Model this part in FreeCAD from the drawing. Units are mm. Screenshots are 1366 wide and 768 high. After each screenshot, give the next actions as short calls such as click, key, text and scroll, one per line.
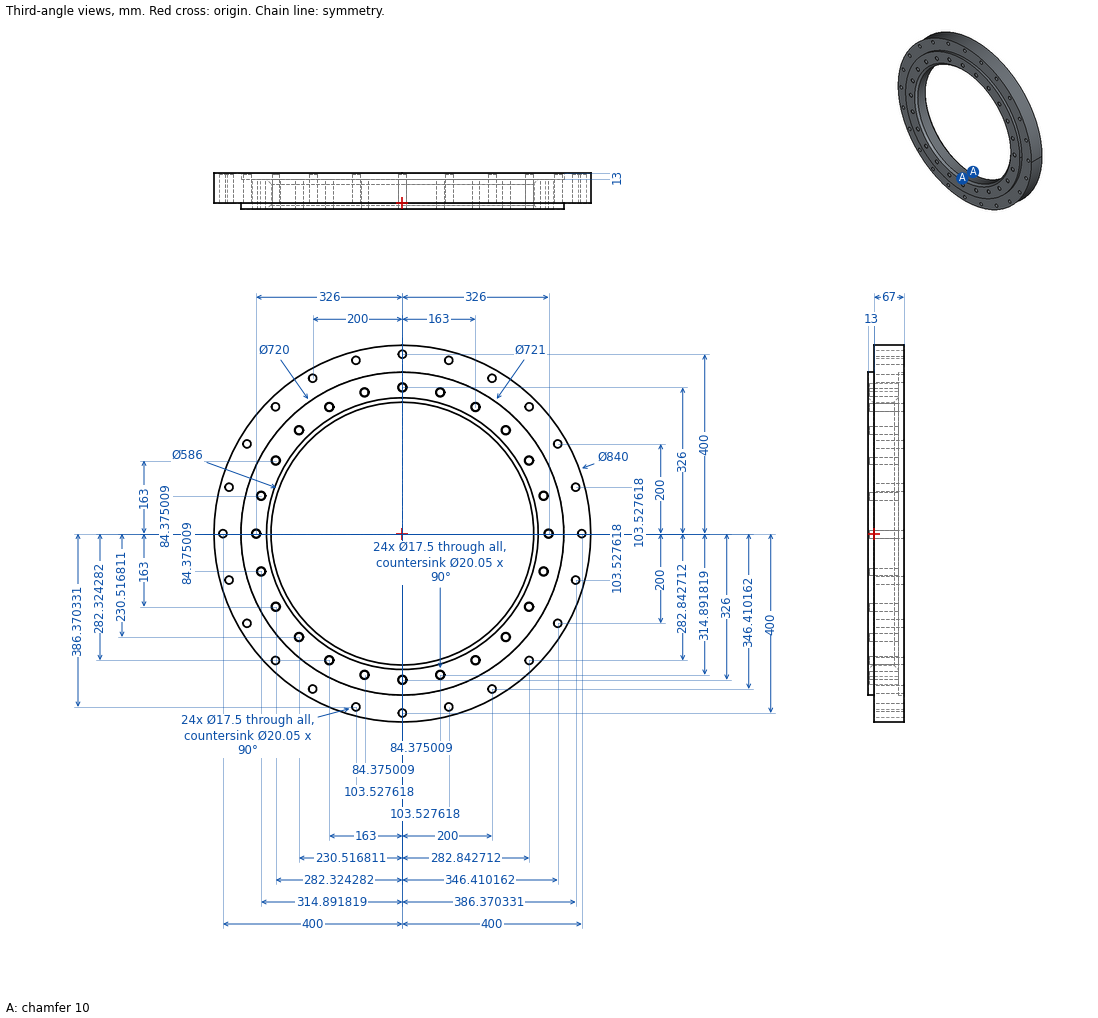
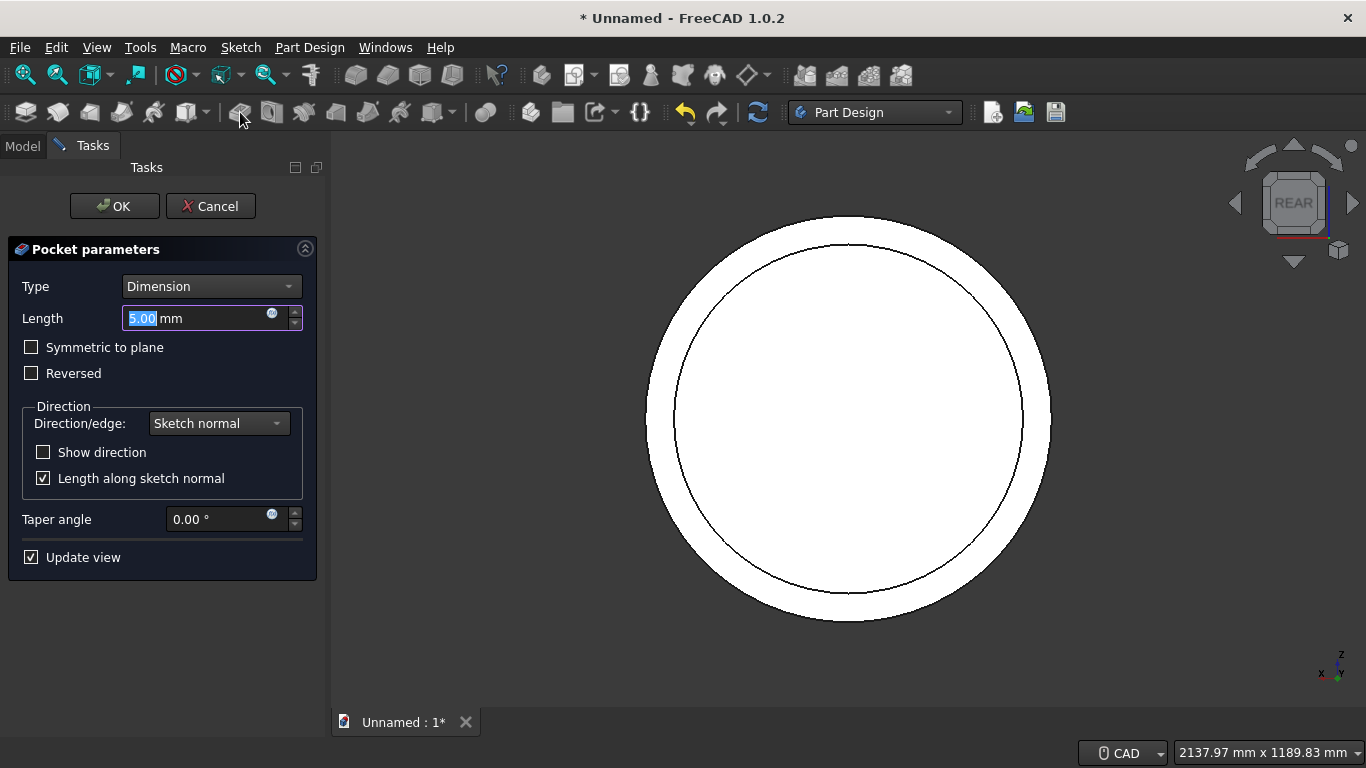
text(13)
key(Tab)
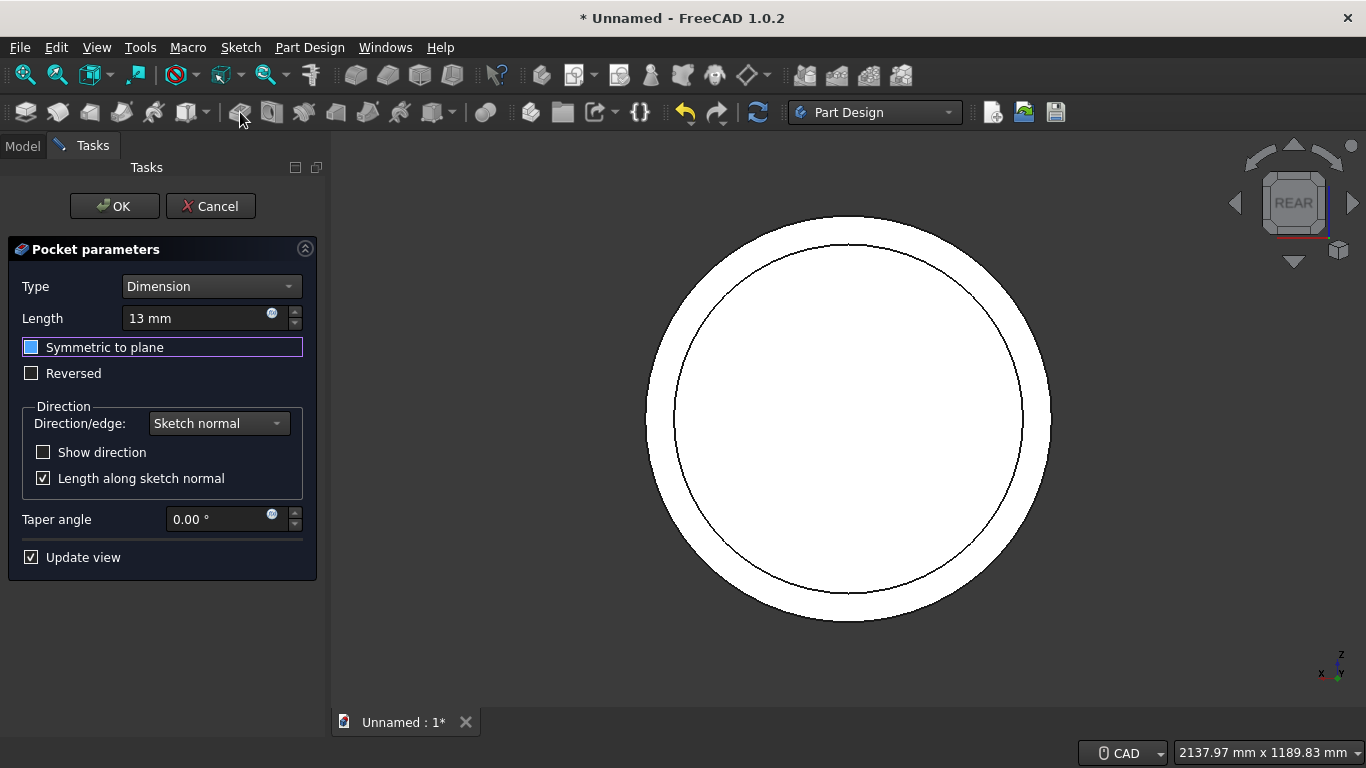
click(115, 206)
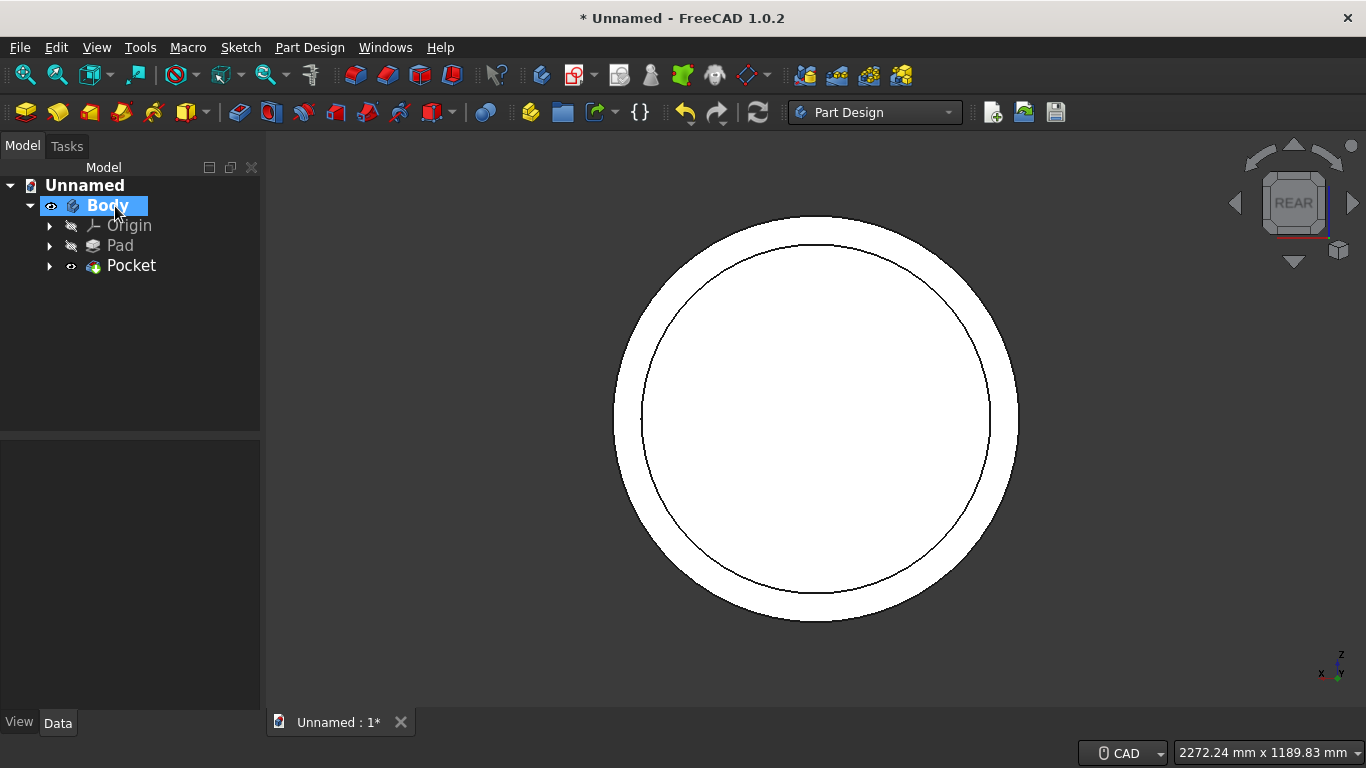
click(574, 76)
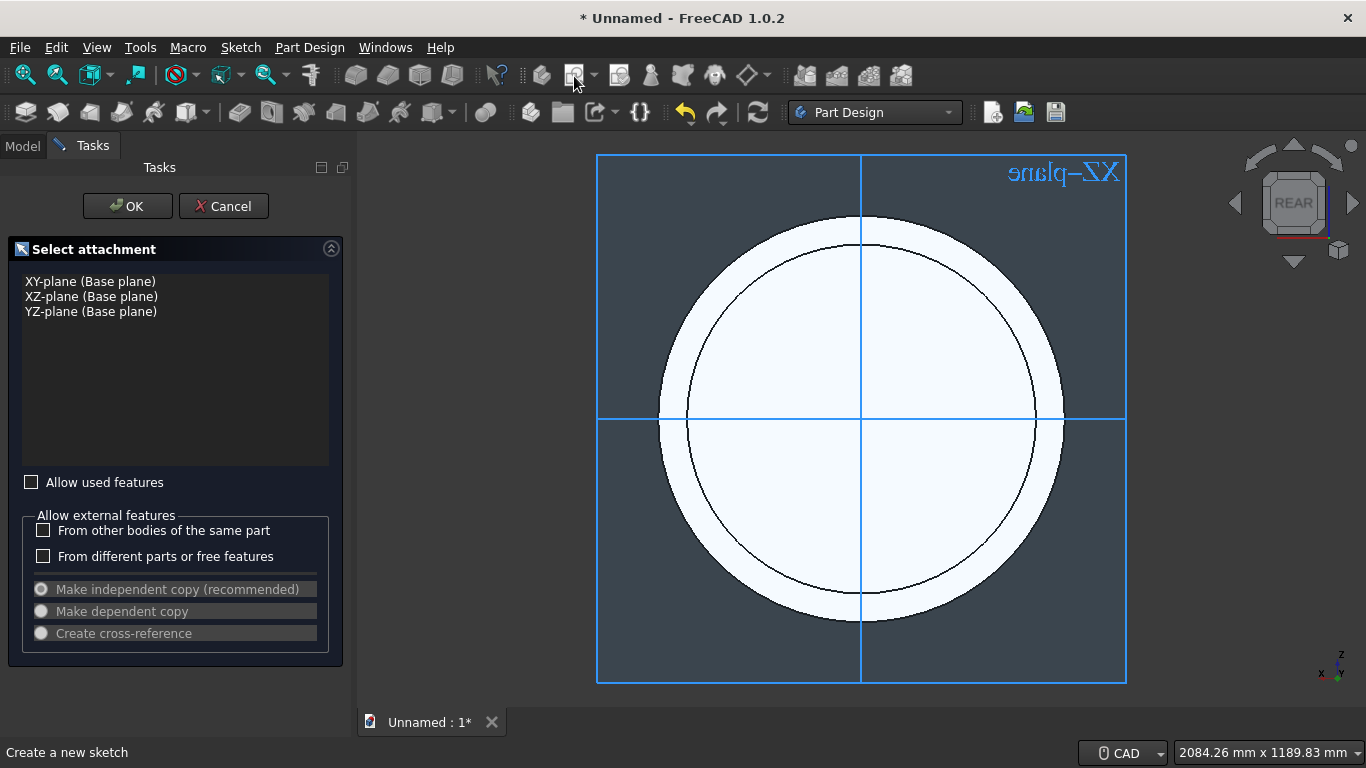
click(82, 296)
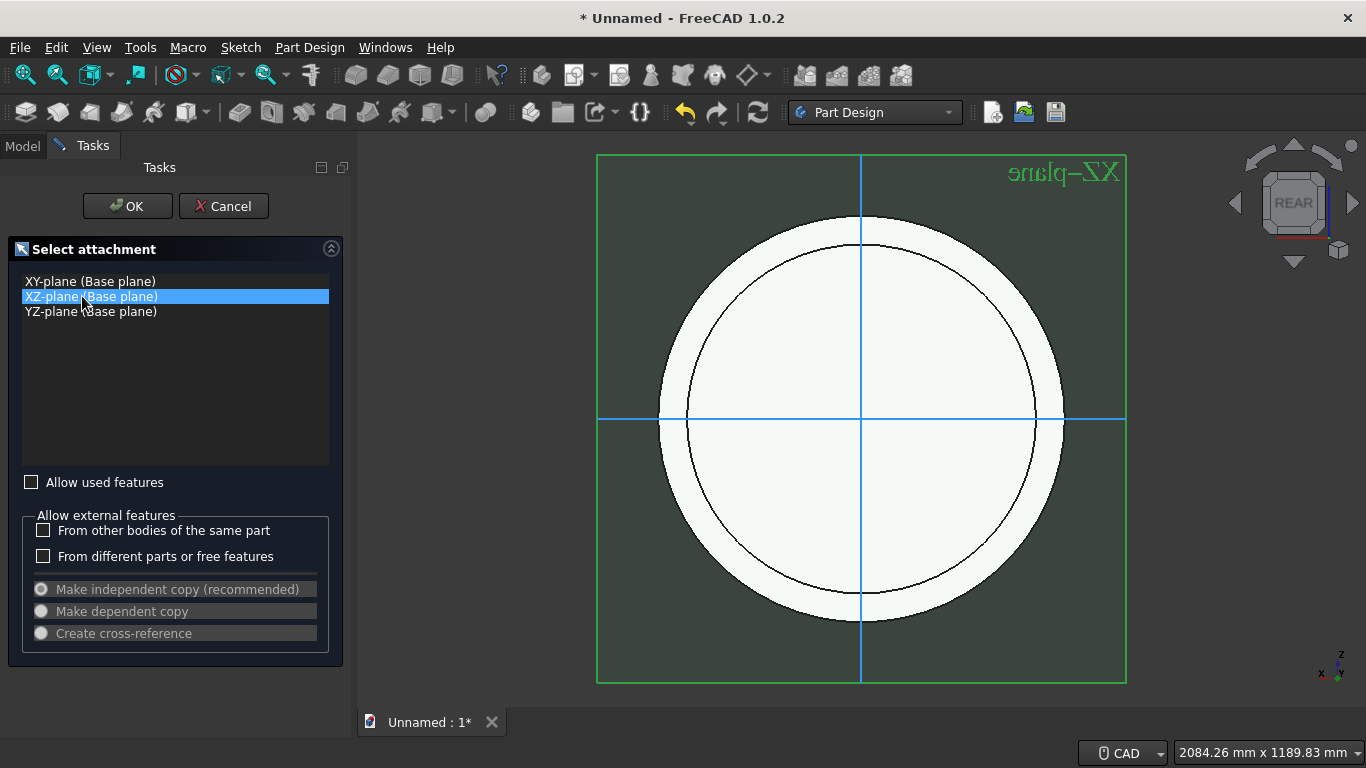
click(128, 206)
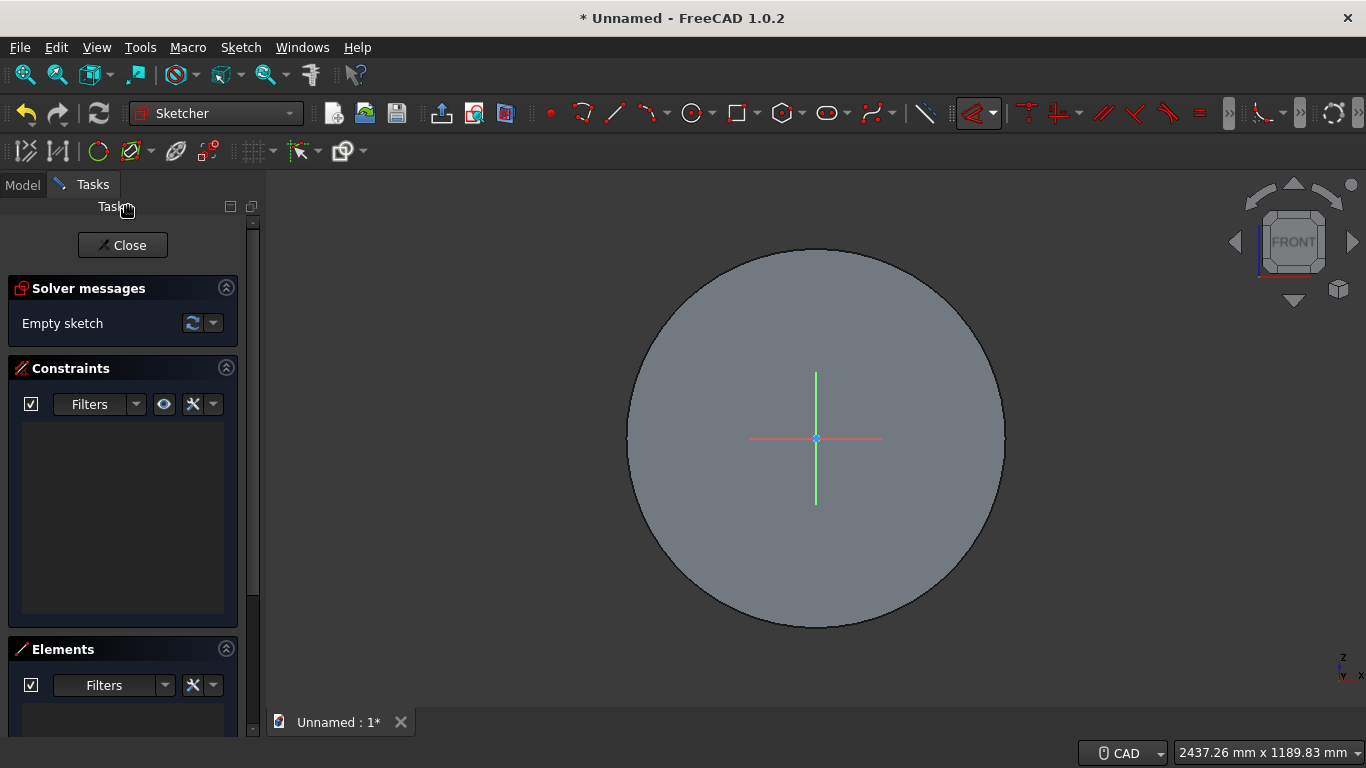
click(692, 114)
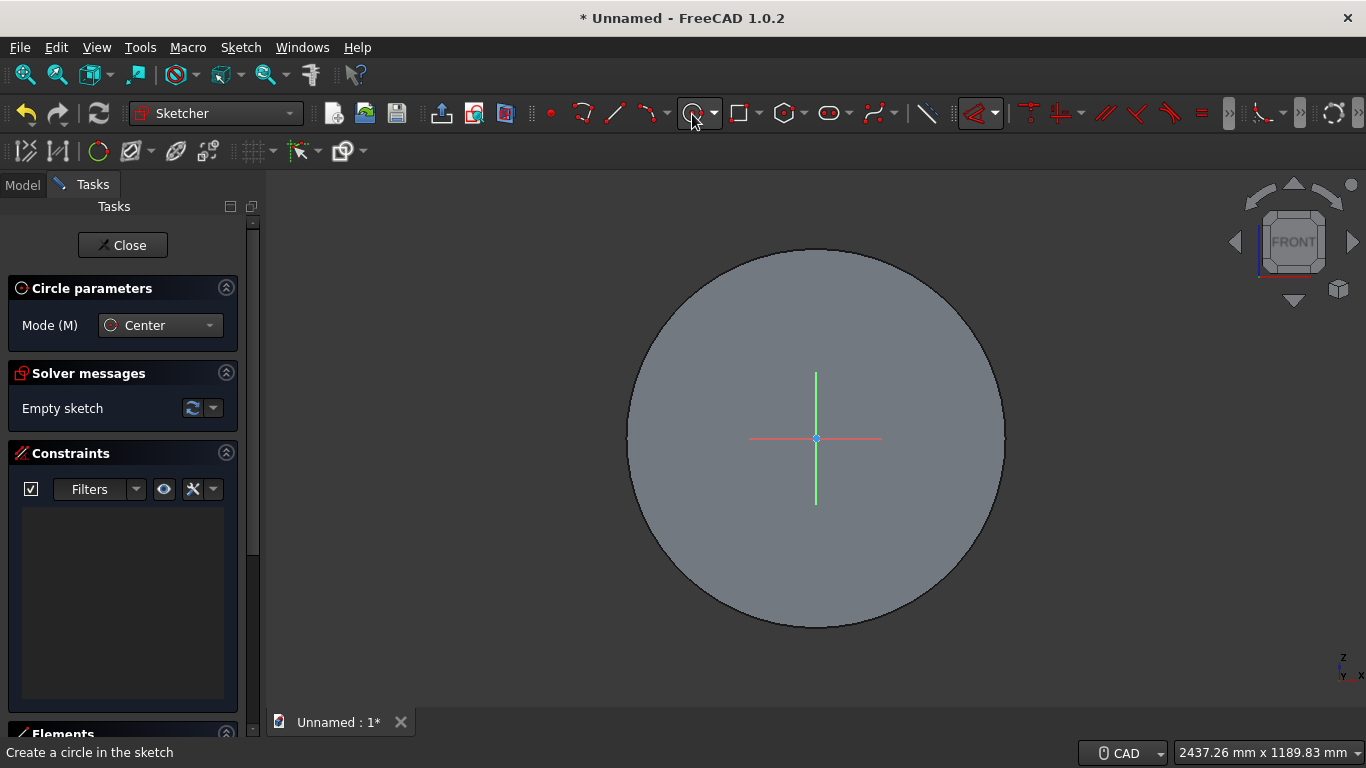
click(816, 439)
click(931, 324)
key(Escape)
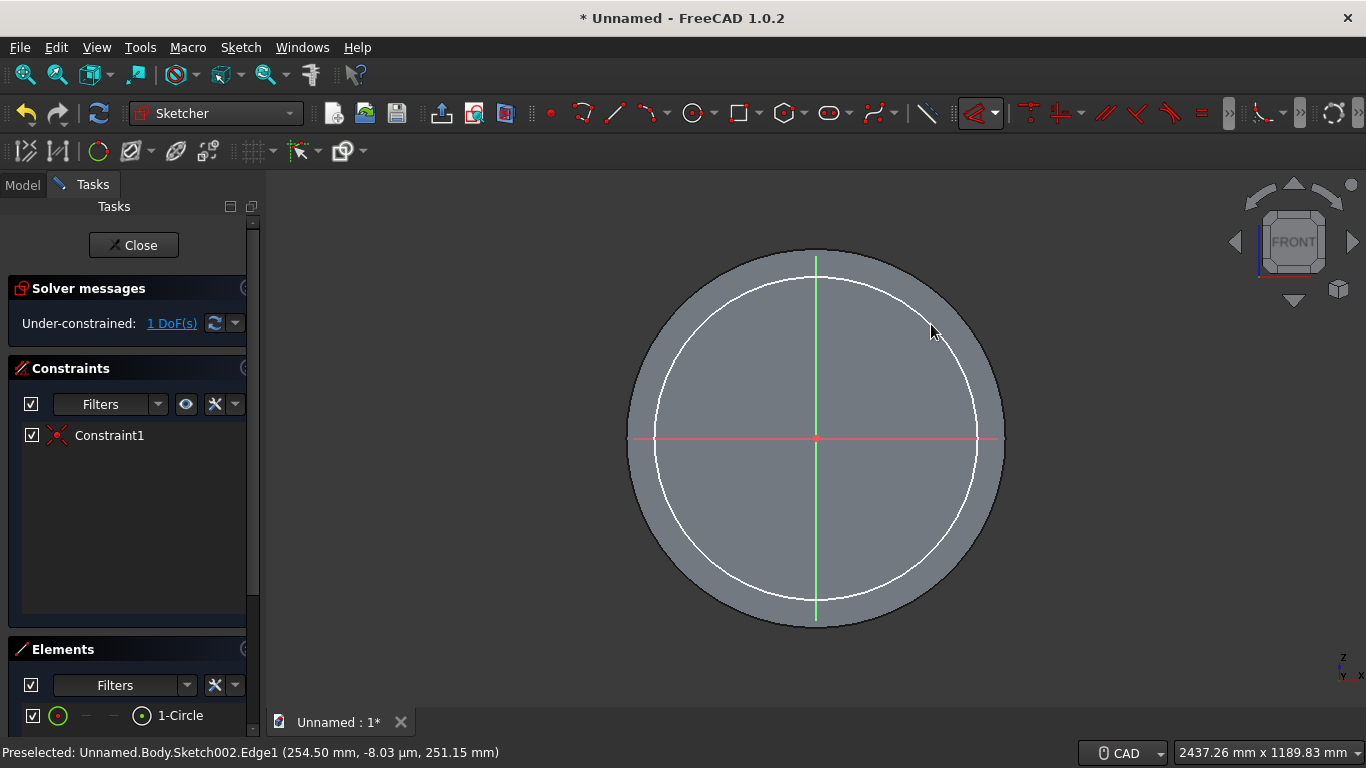
click(930, 324)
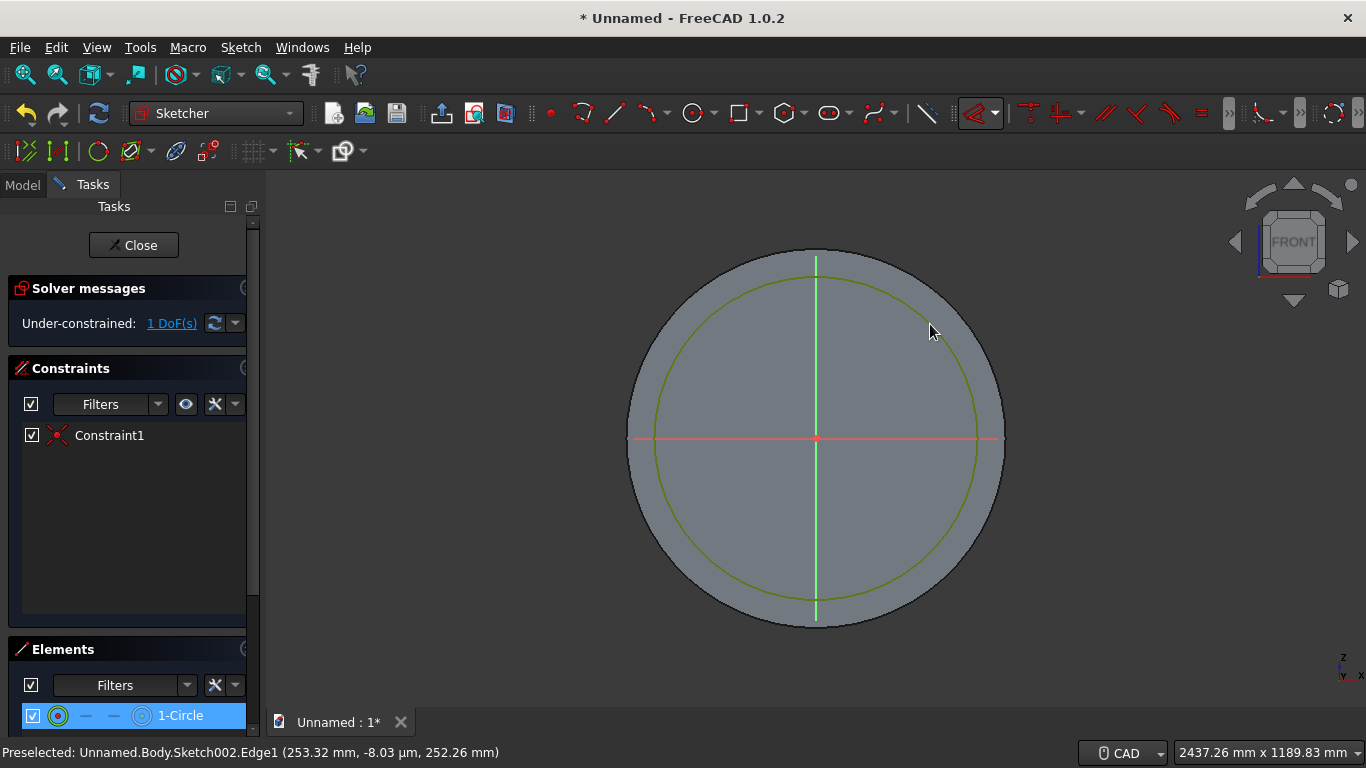
key(k)
key(o)